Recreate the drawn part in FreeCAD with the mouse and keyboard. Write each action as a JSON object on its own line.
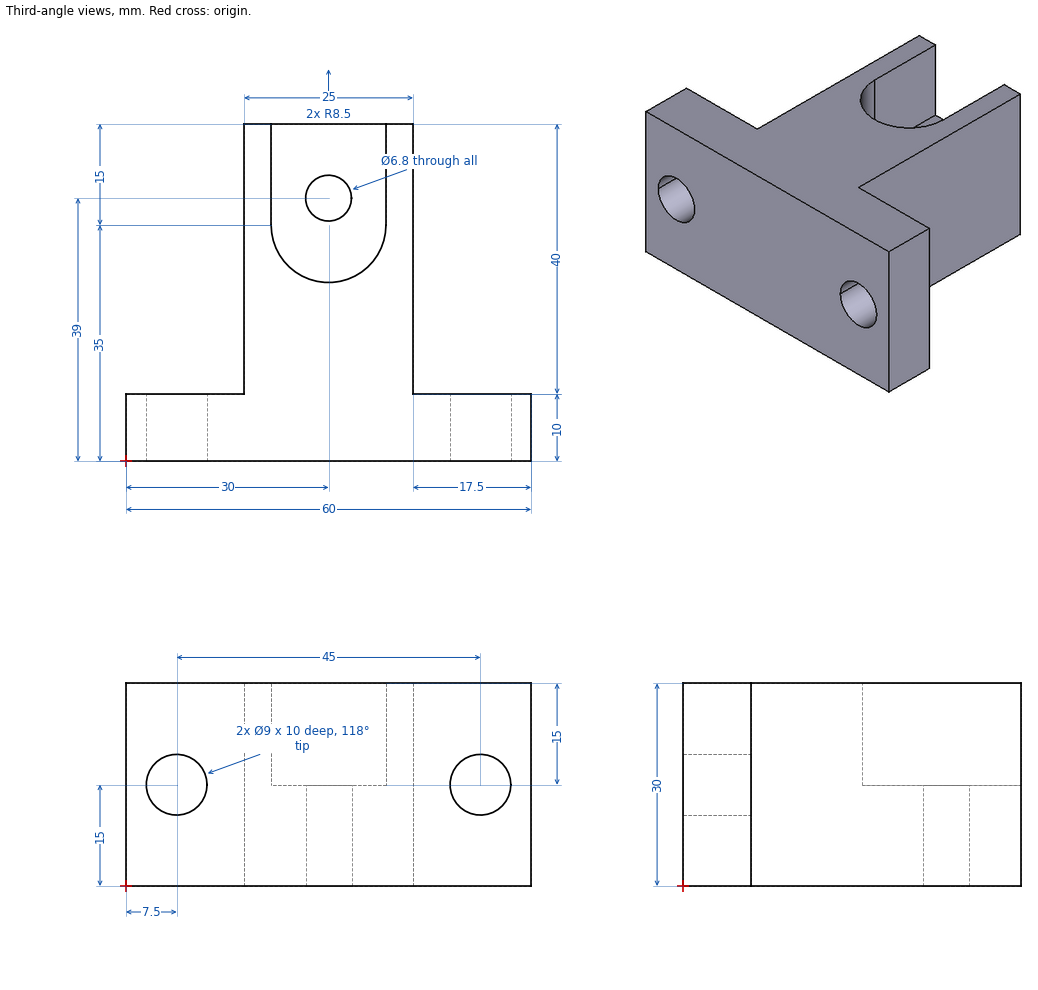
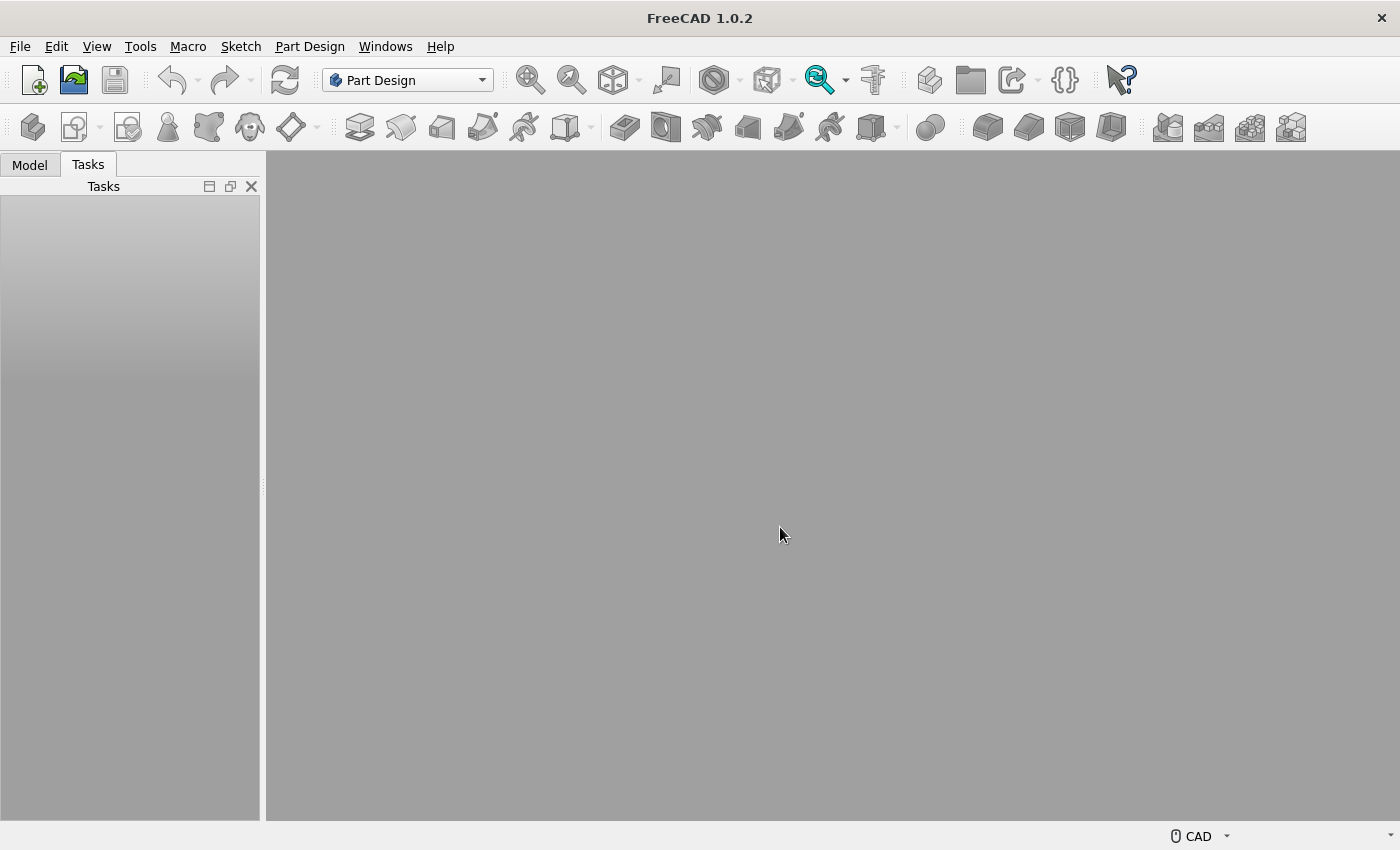
{"action": "key", "text": "ctrl+n"}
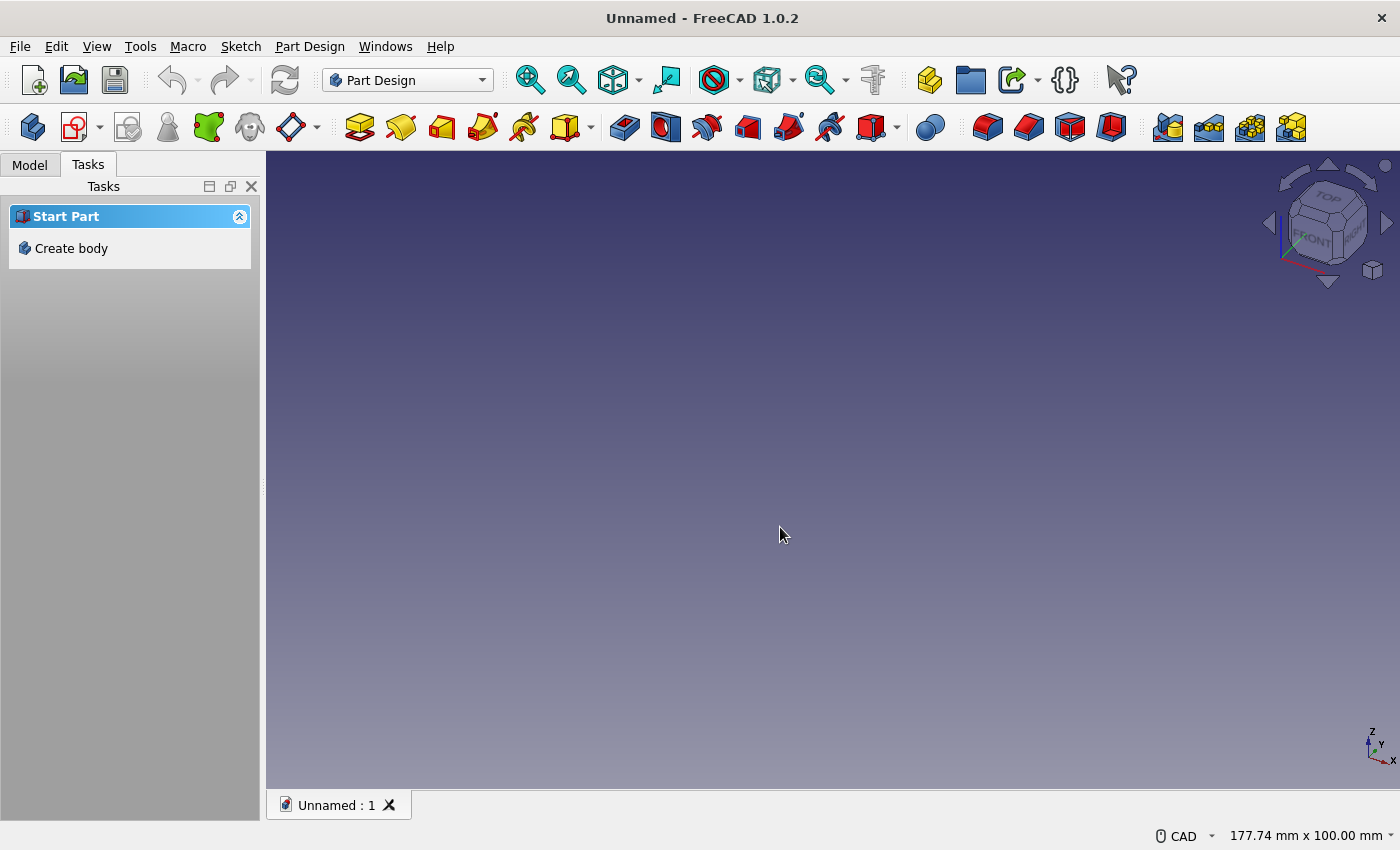
{"action": "left_click", "coordinate": [74, 128]}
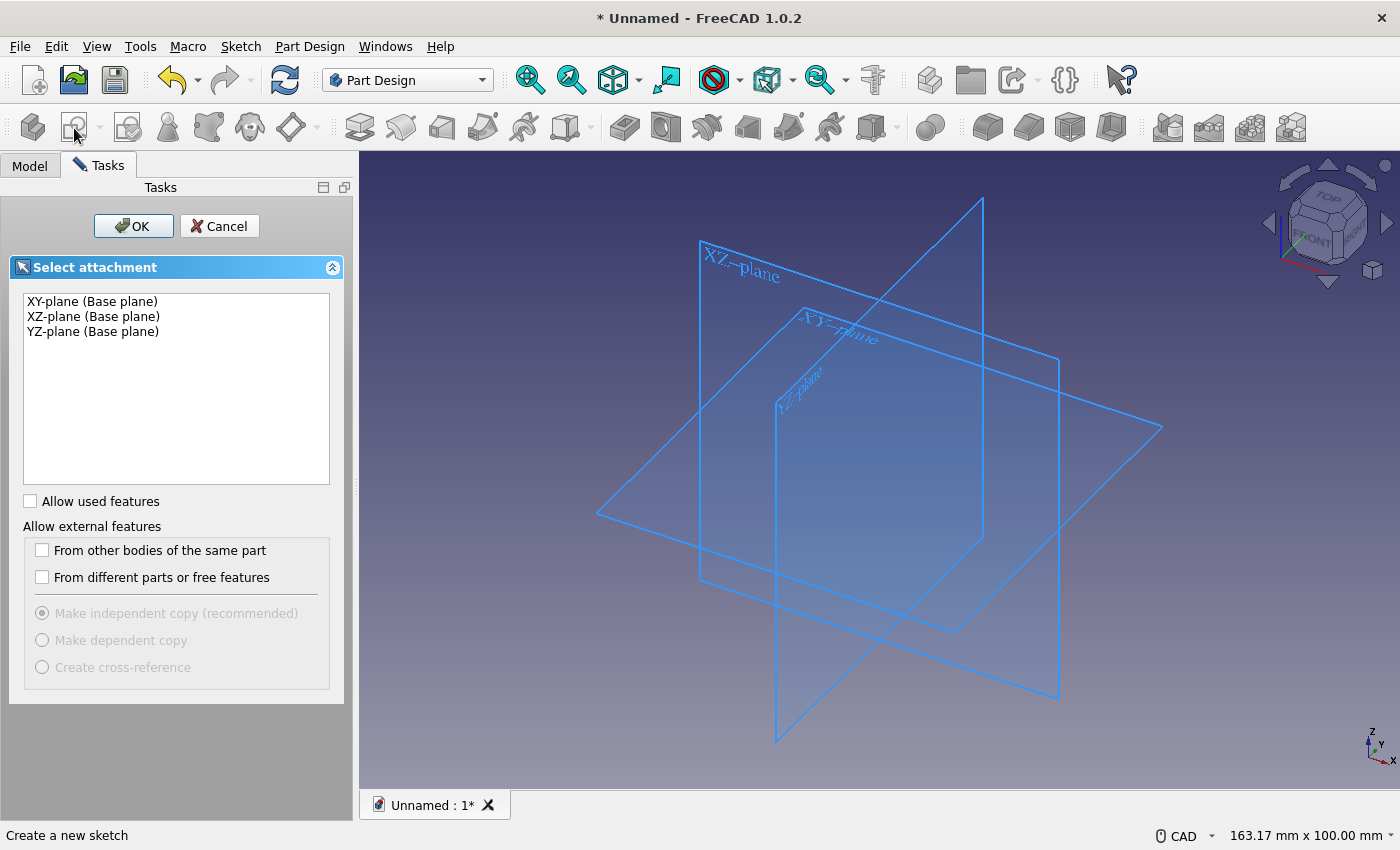
{"action": "left_click", "coordinate": [84, 302]}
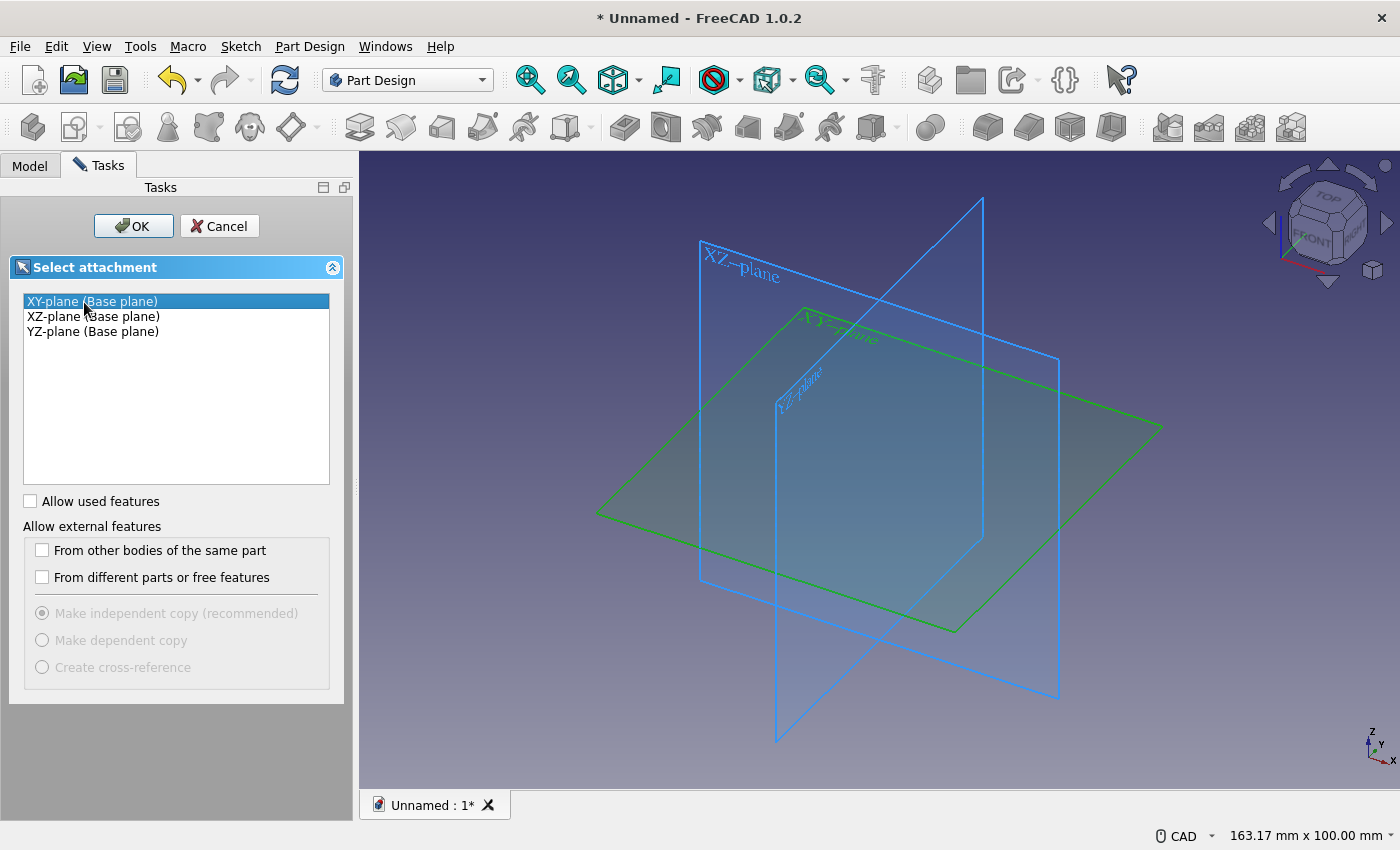
{"action": "left_click", "coordinate": [134, 226]}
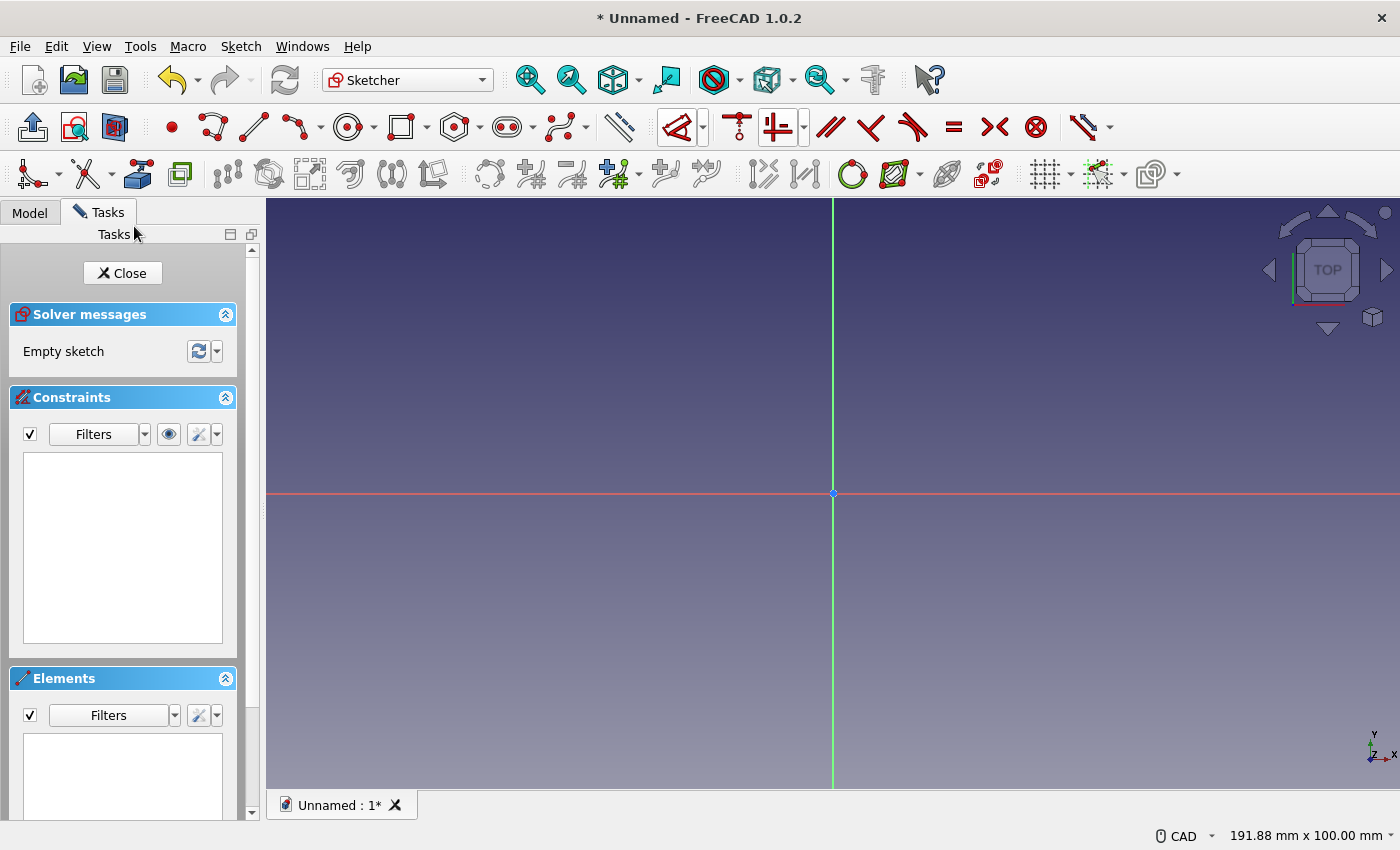
{"action": "scroll", "coordinate": [294, 761], "scroll_direction": "down", "scroll_amount": 1}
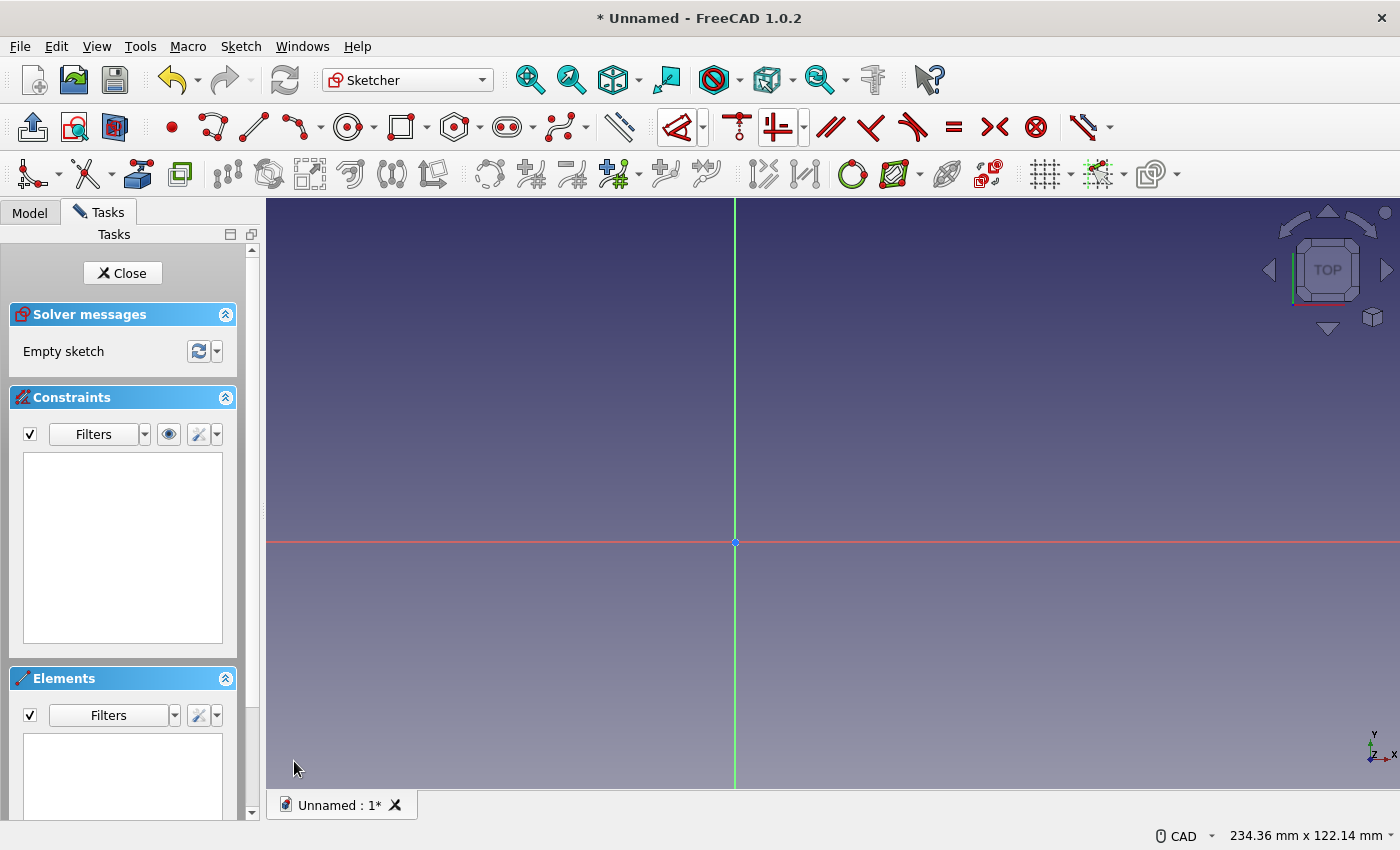
{"action": "scroll", "coordinate": [1116, 274], "scroll_direction": "up", "scroll_amount": 2}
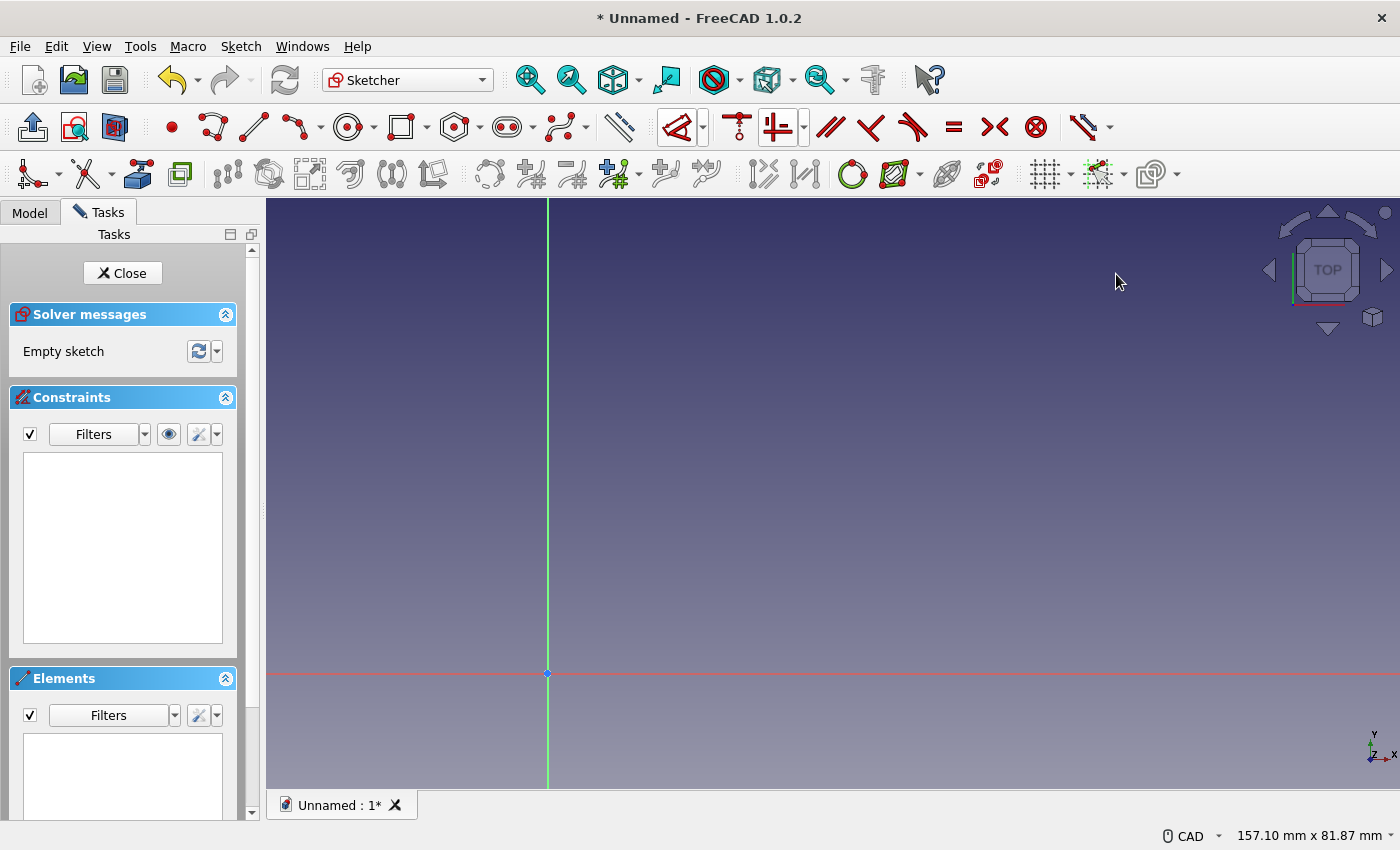
{"action": "left_click", "coordinate": [213, 128]}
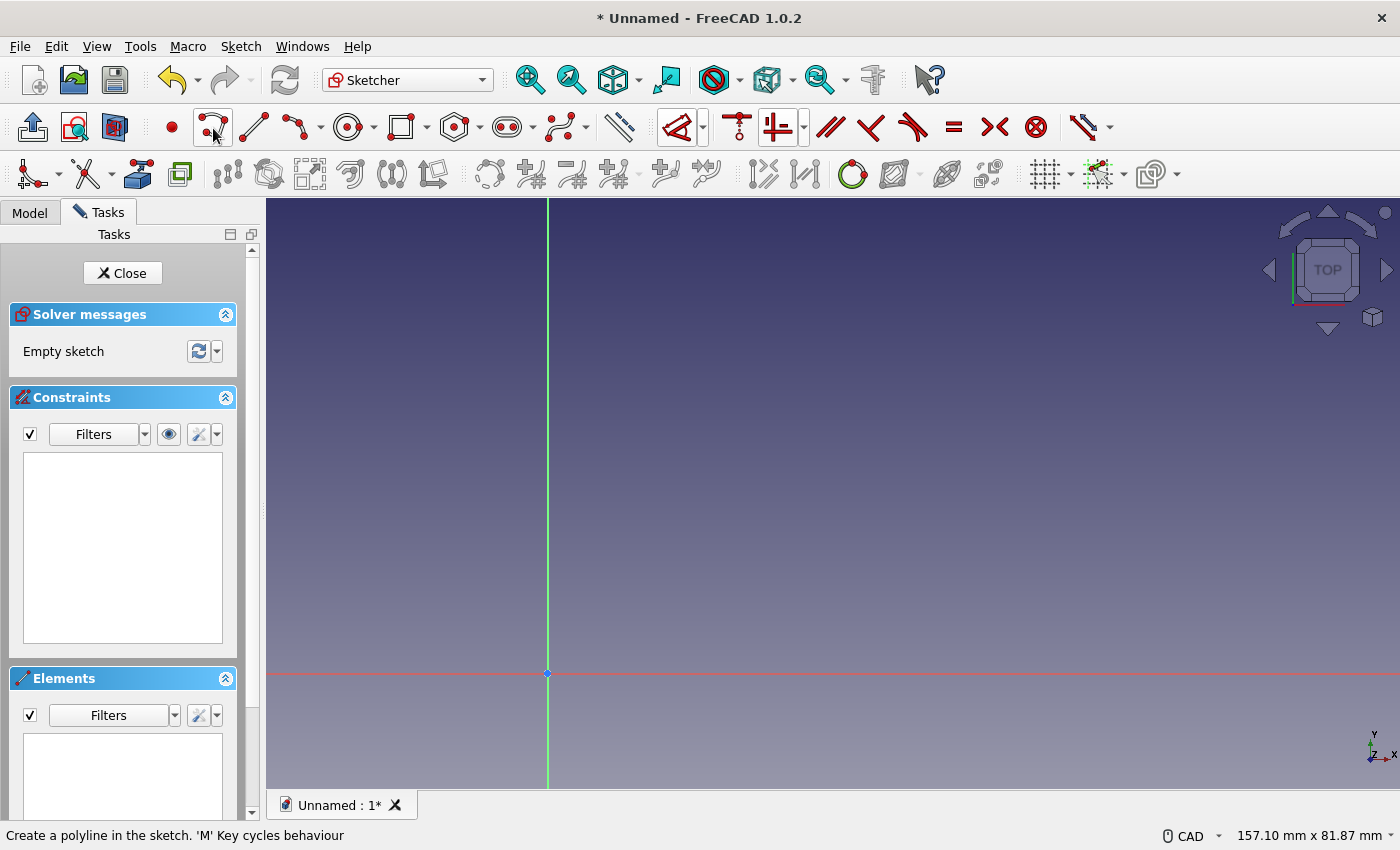
{"action": "left_click", "coordinate": [548, 674]}
{"action": "left_click", "coordinate": [981, 665]}
{"action": "left_click", "coordinate": [981, 602]}
{"action": "left_click", "coordinate": [854, 602]}
{"action": "left_click", "coordinate": [854, 313]}
{"action": "left_click", "coordinate": [674, 313]}
{"action": "left_click", "coordinate": [674, 602]}
{"action": "left_click", "coordinate": [557, 602]}
{"action": "left_click", "coordinate": [548, 674]}
{"action": "key", "text": "Escape"}
{"action": "key", "text": "Escape"}